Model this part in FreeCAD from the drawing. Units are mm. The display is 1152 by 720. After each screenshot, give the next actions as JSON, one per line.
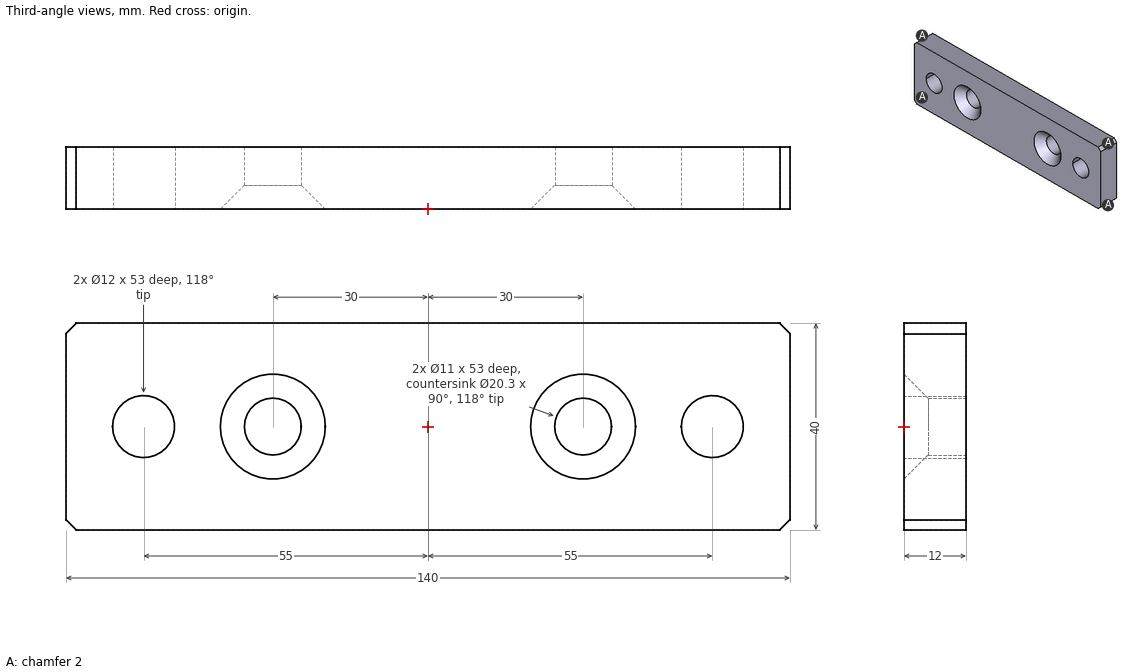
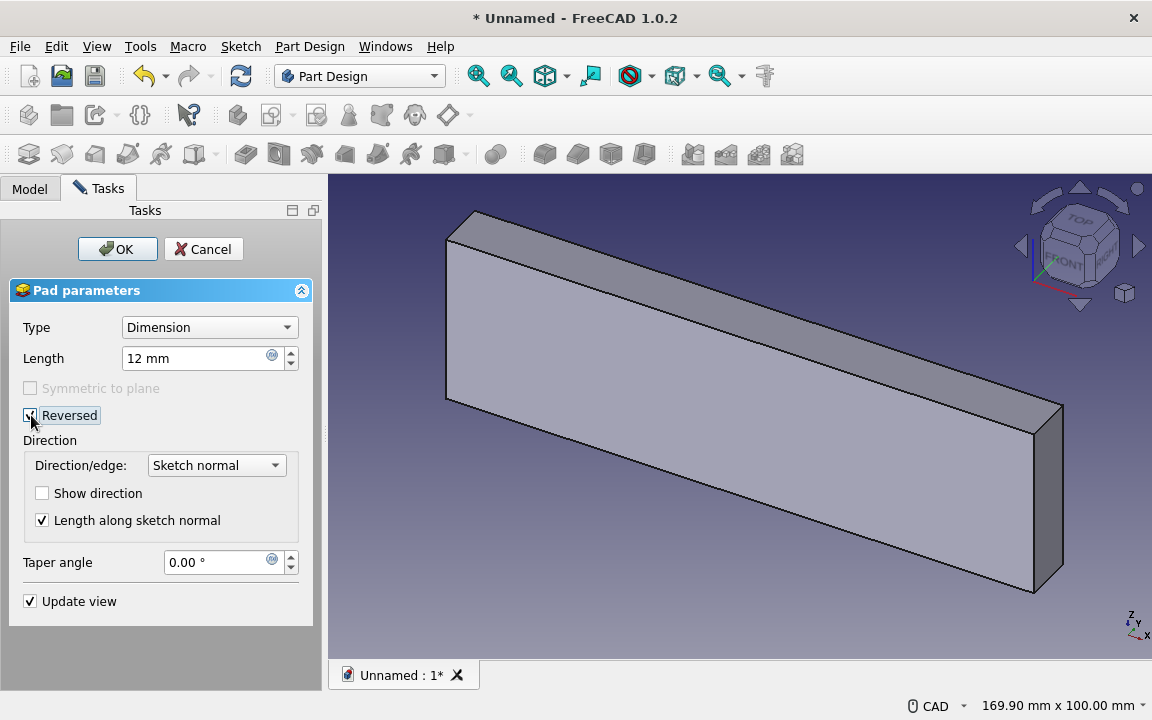
{"action": "left_click", "coordinate": [118, 249]}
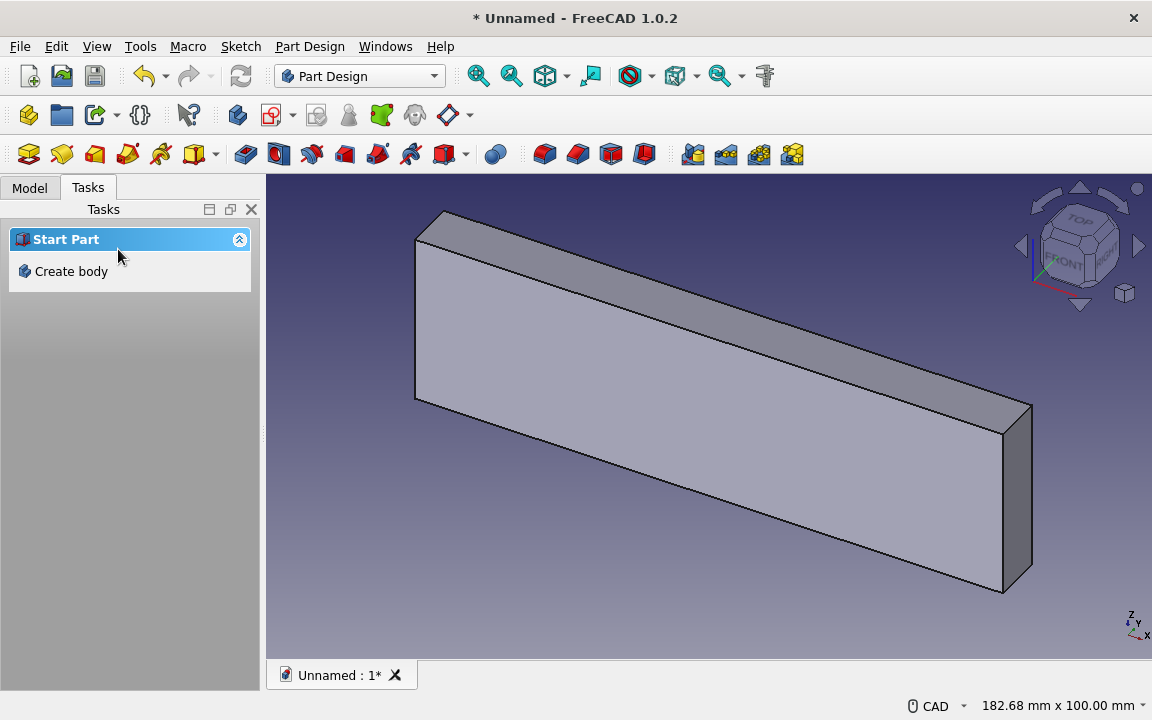
{"action": "key", "text": "4"}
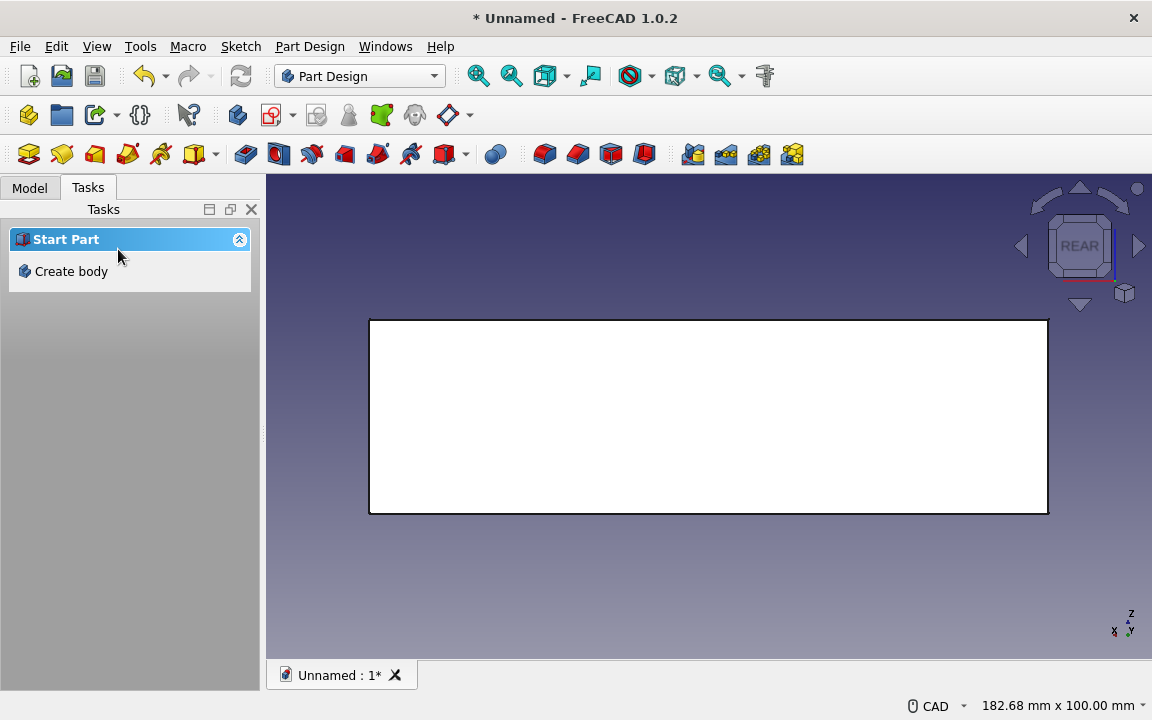
{"action": "left_click", "coordinate": [515, 415]}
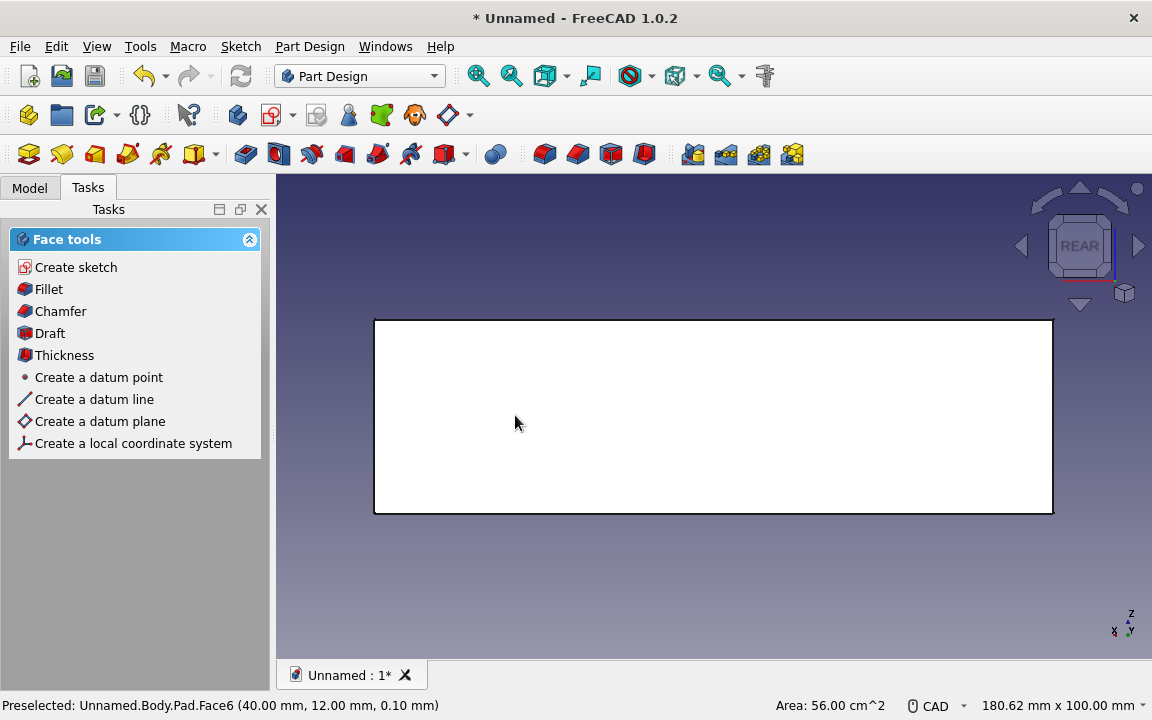
{"action": "left_click", "coordinate": [270, 116]}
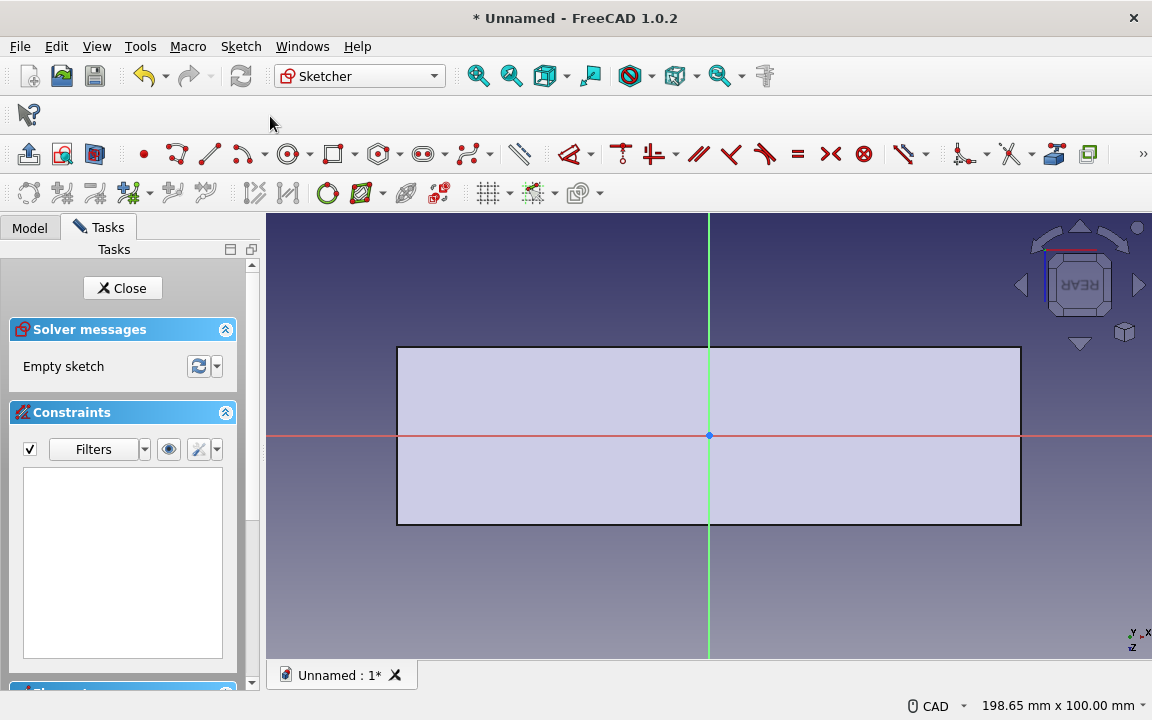
{"action": "scroll", "coordinate": [331, 436], "scroll_direction": "down", "scroll_amount": 1}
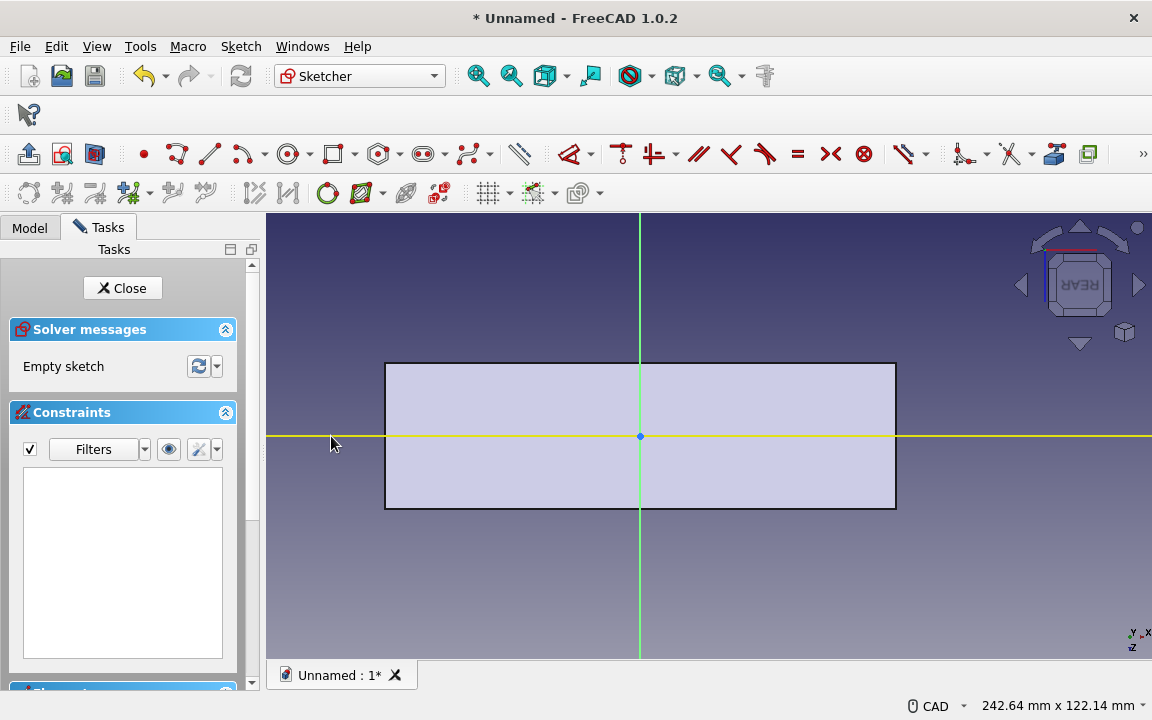
{"action": "key", "text": "g c"}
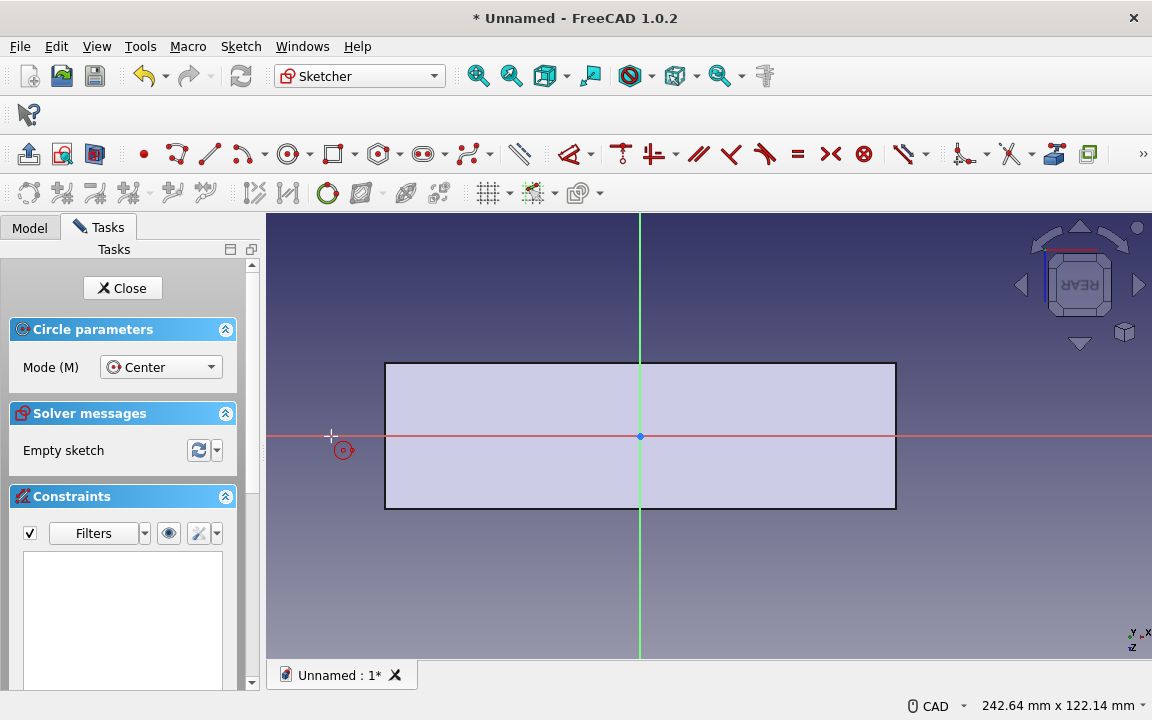
{"action": "left_click", "coordinate": [440, 436]}
{"action": "mouse_move", "coordinate": [455, 421]}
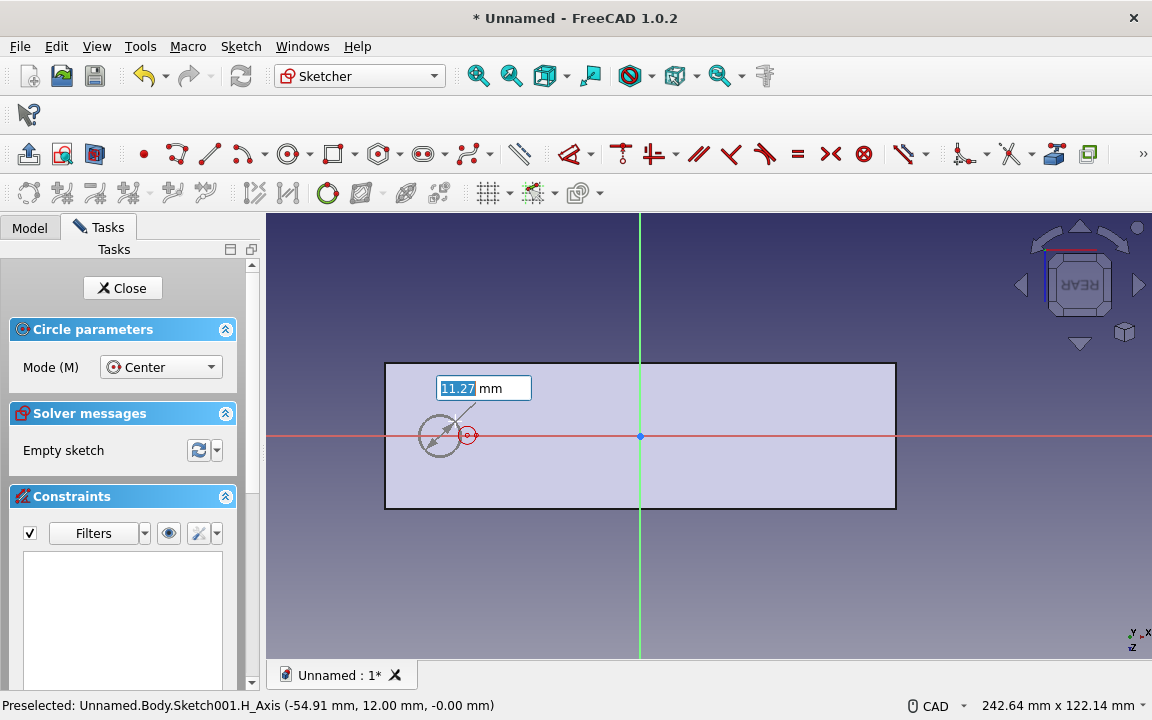
{"action": "type", "text": "12"}
{"action": "key", "text": "Return"}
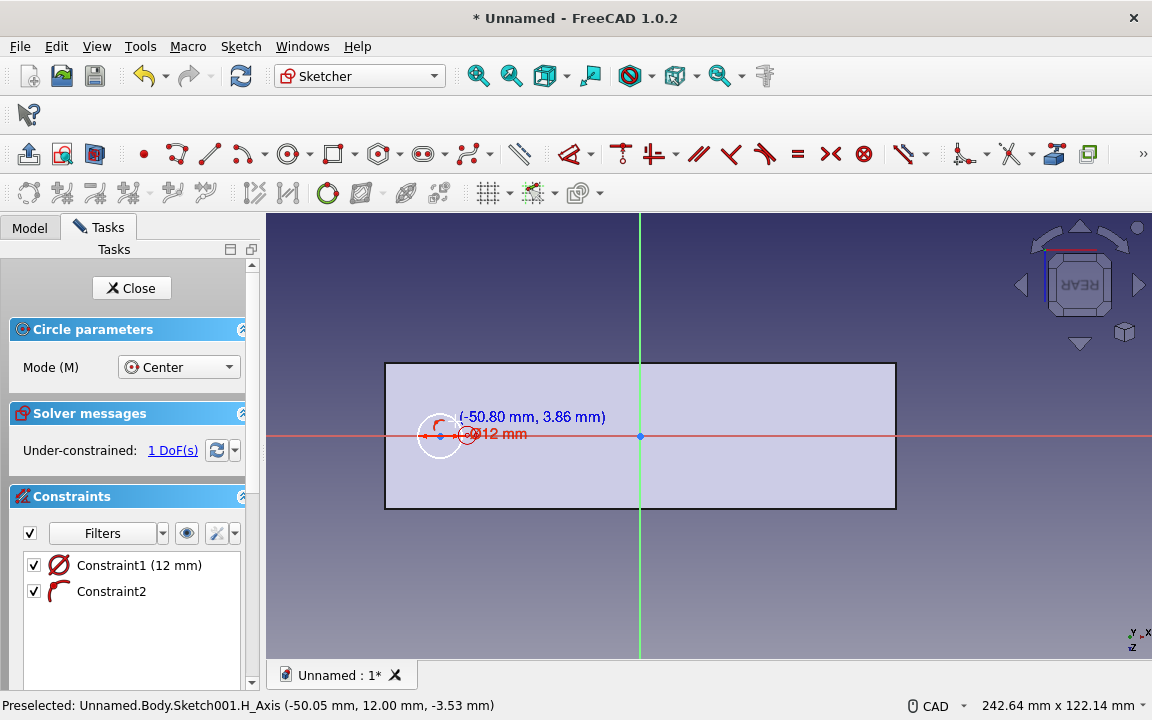
{"action": "left_click", "coordinate": [841, 436]}
{"action": "mouse_move", "coordinate": [857, 421]}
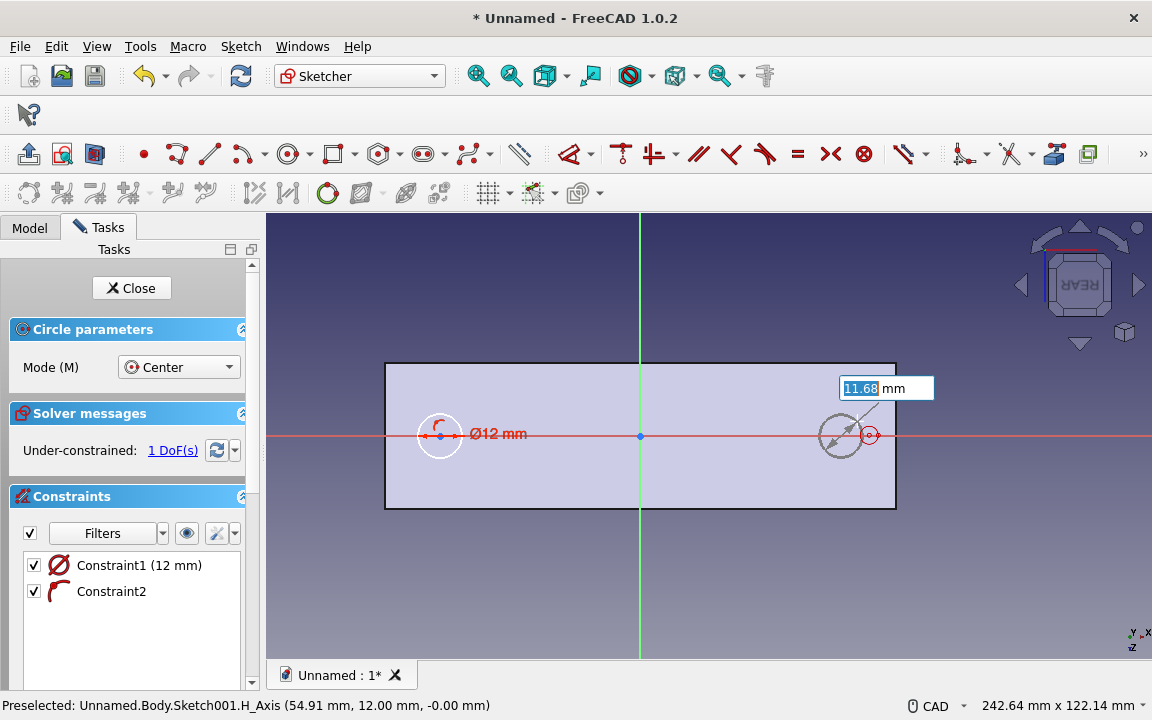
{"action": "type", "text": "12"}
{"action": "key", "text": "Return"}
{"action": "key", "text": "Escape"}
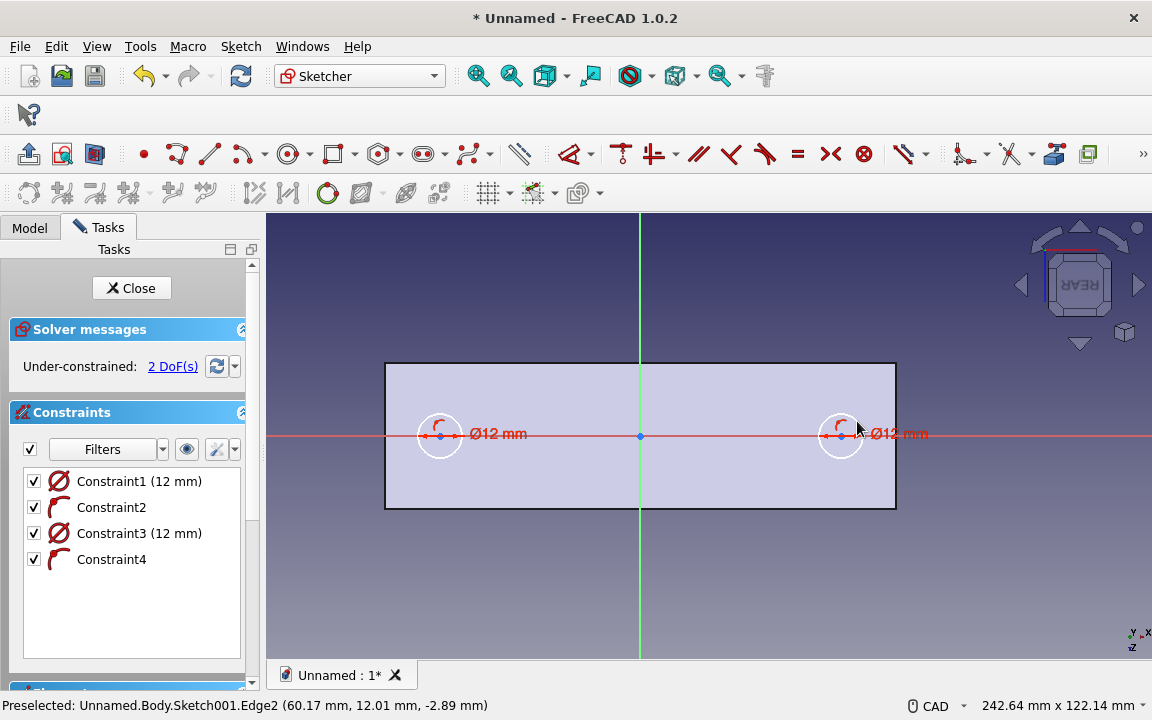
{"action": "key", "text": "d"}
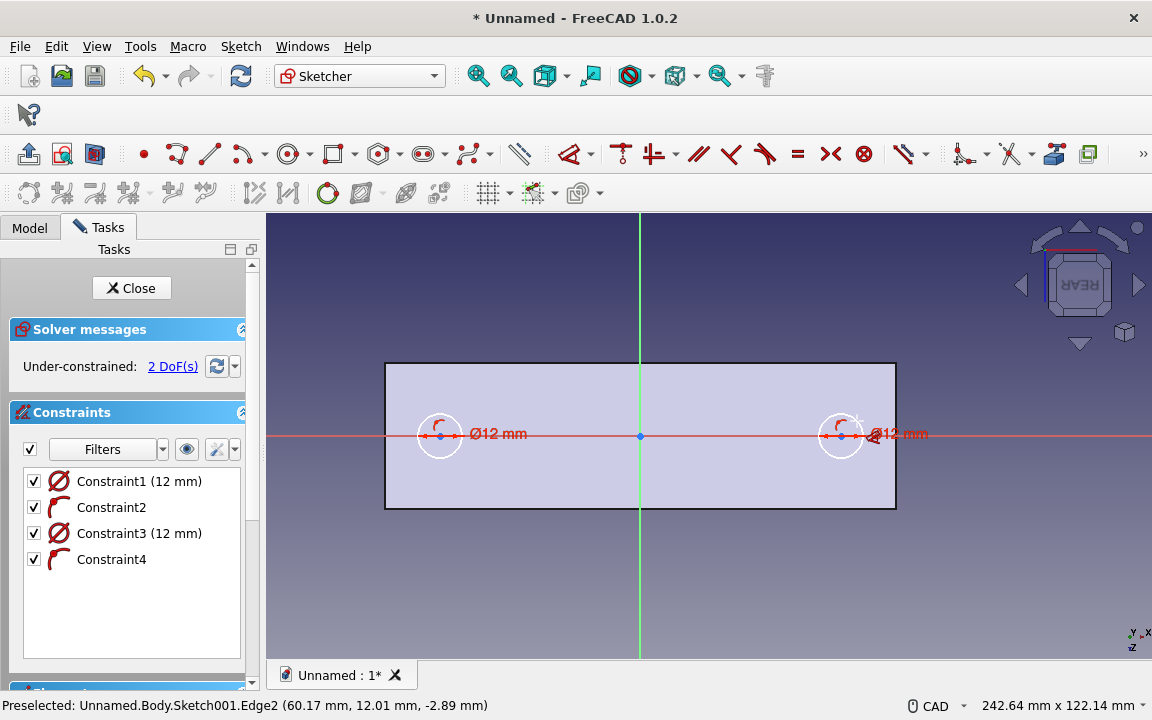
{"action": "left_click", "coordinate": [440, 436]}
{"action": "left_click", "coordinate": [540, 470]}